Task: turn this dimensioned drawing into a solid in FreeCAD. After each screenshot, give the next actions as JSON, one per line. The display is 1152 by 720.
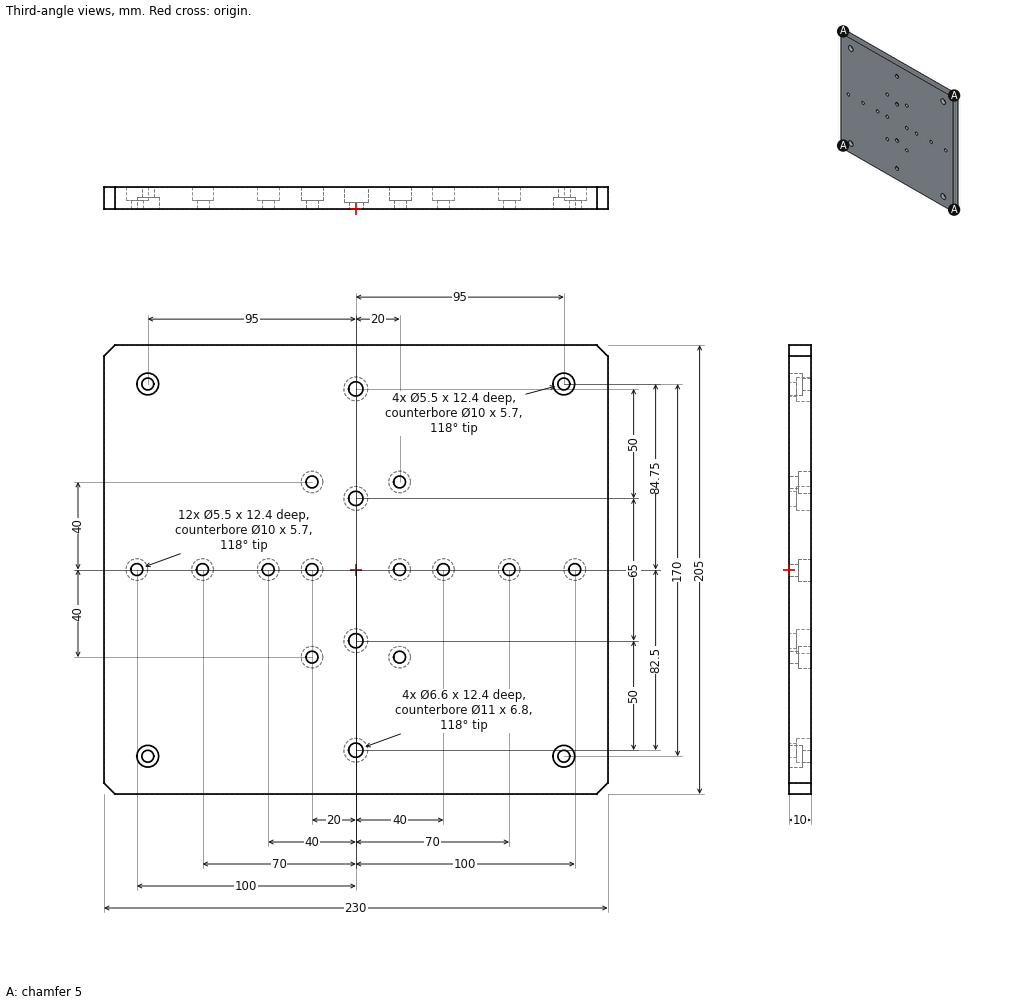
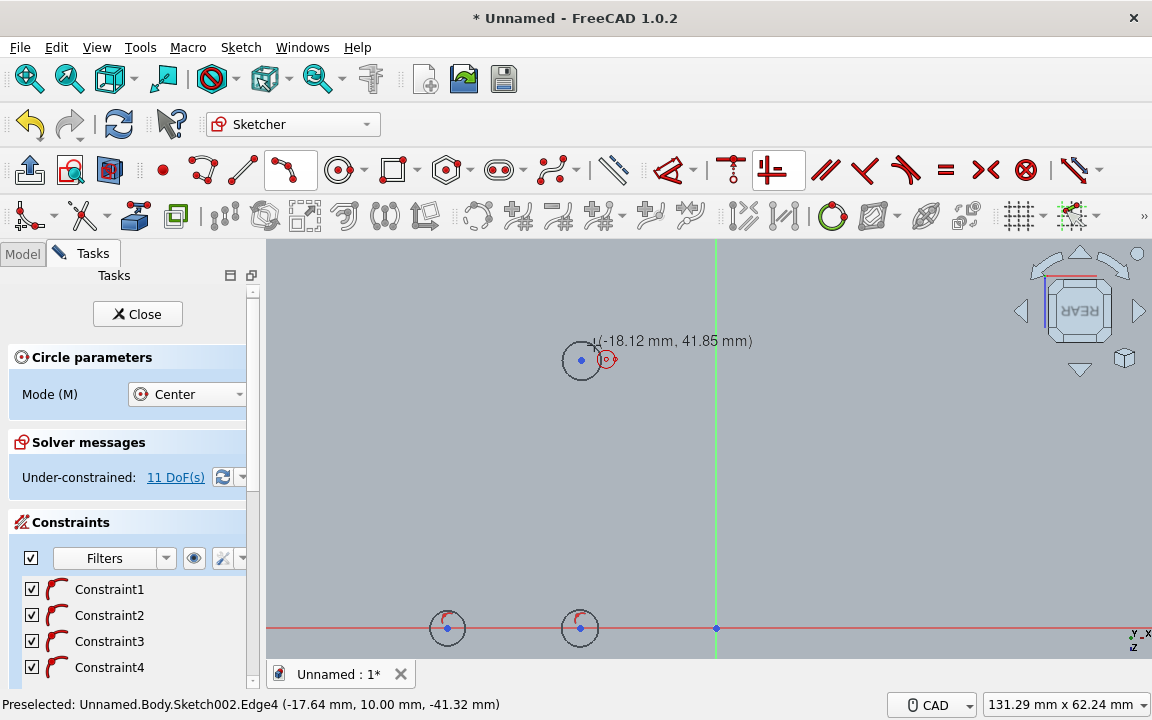
{"action": "scroll", "coordinate": [596, 345], "scroll_direction": "down", "scroll_amount": 5}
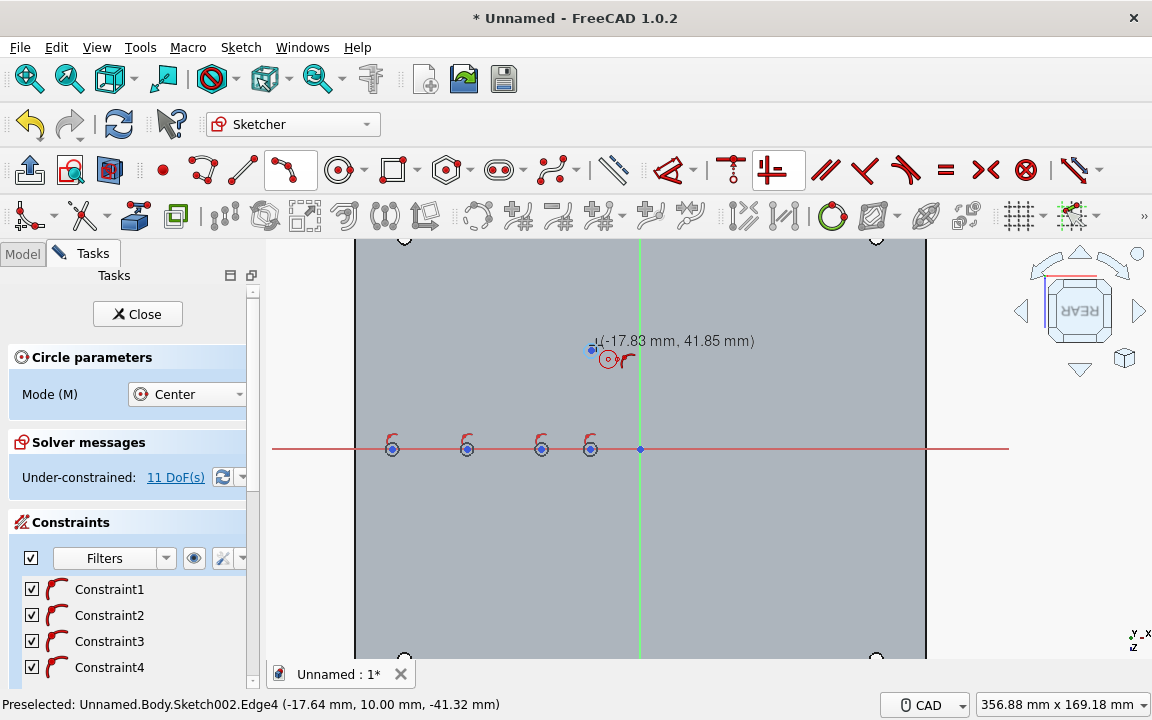
{"action": "scroll", "coordinate": [591, 549], "scroll_direction": "up", "scroll_amount": 7}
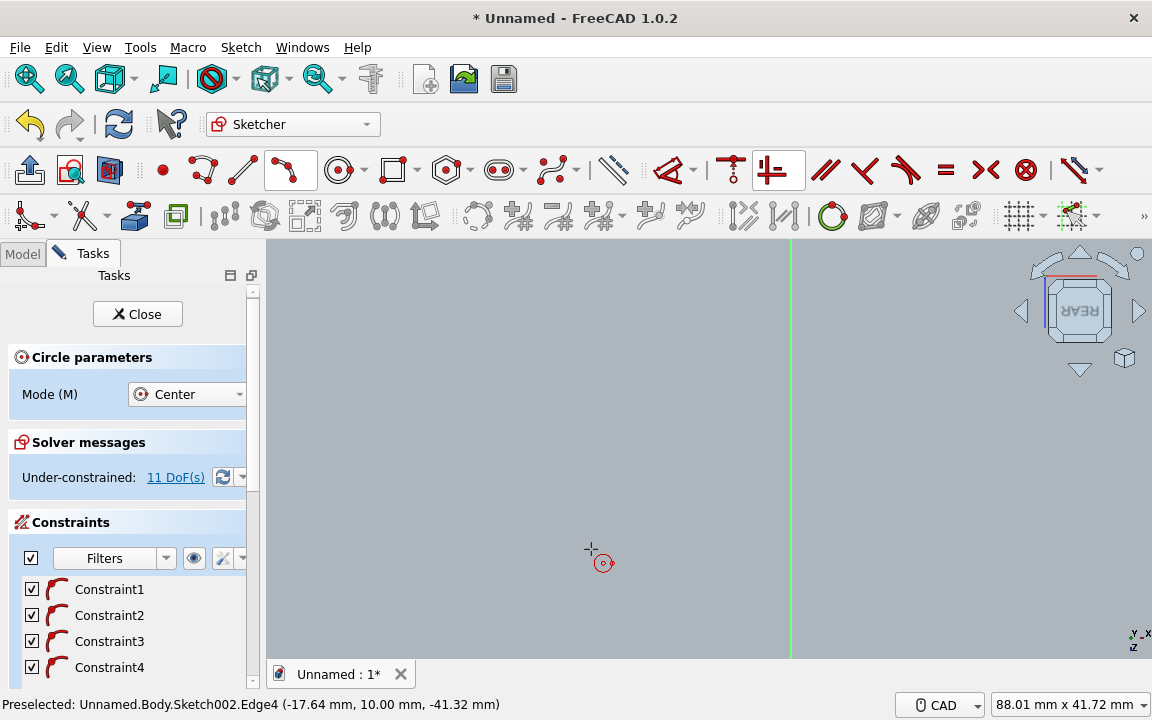
{"action": "scroll", "coordinate": [591, 549], "scroll_direction": "down", "scroll_amount": 7}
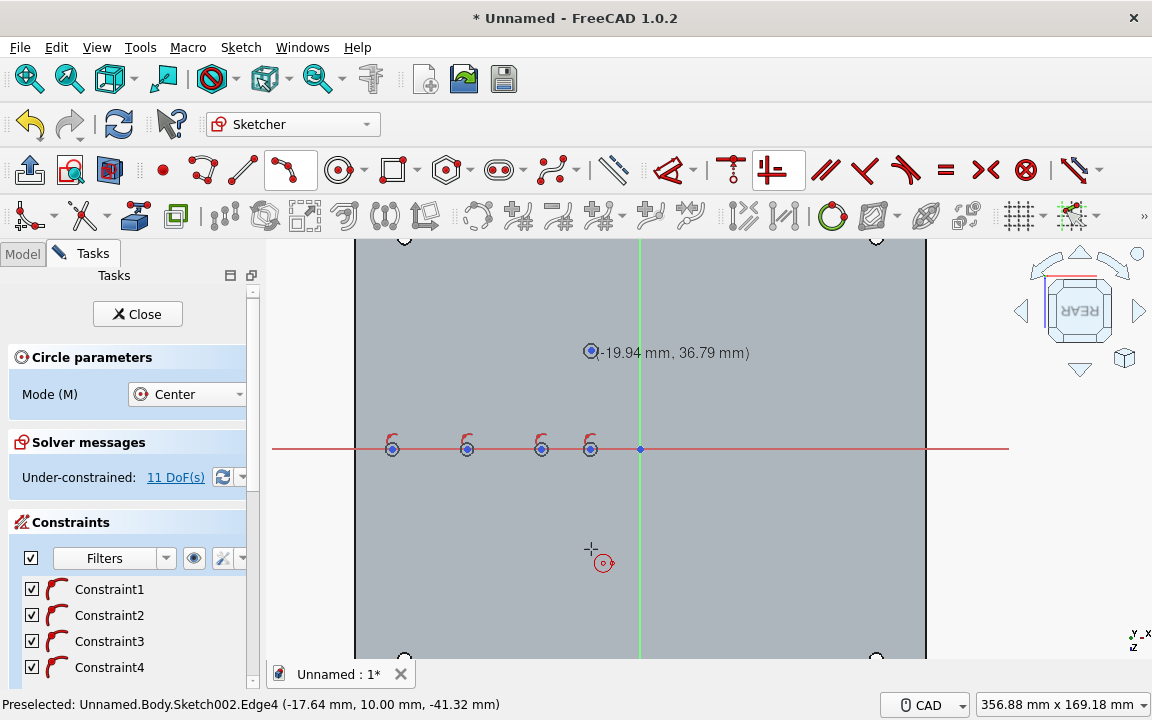
{"action": "left_click", "coordinate": [591, 549]}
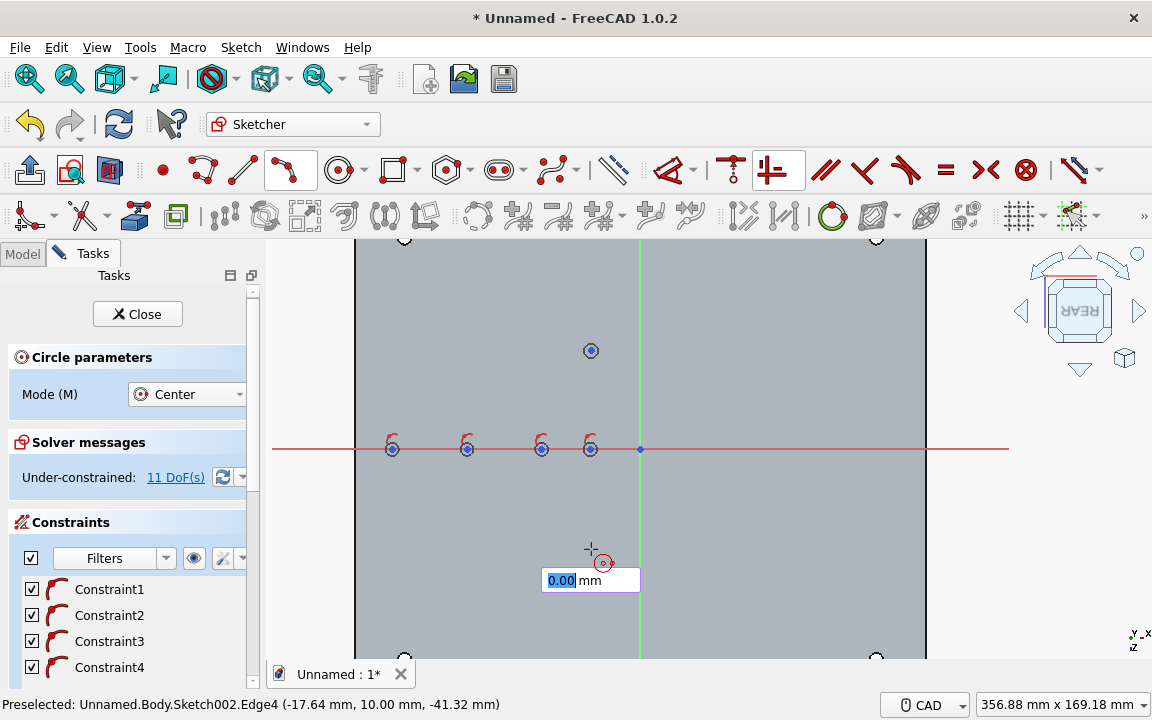
{"action": "scroll", "coordinate": [596, 544], "scroll_direction": "up", "scroll_amount": 5}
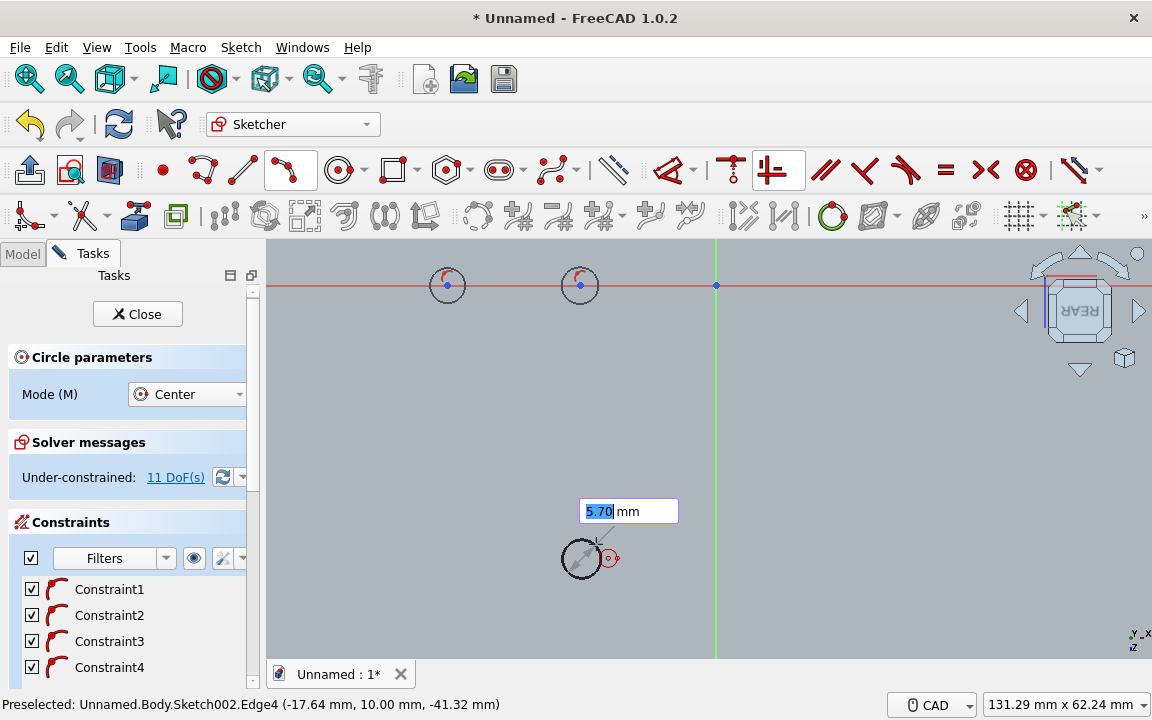
{"action": "left_click", "coordinate": [594, 542]}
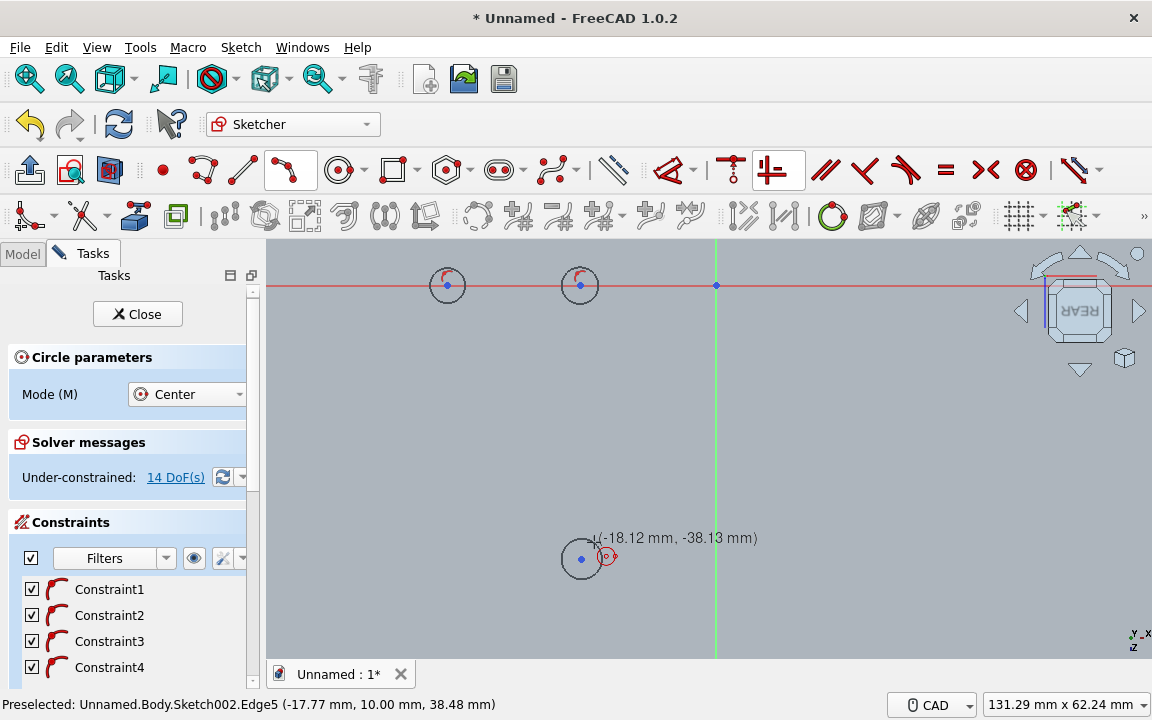
{"action": "scroll", "coordinate": [851, 556], "scroll_direction": "up", "scroll_amount": 2}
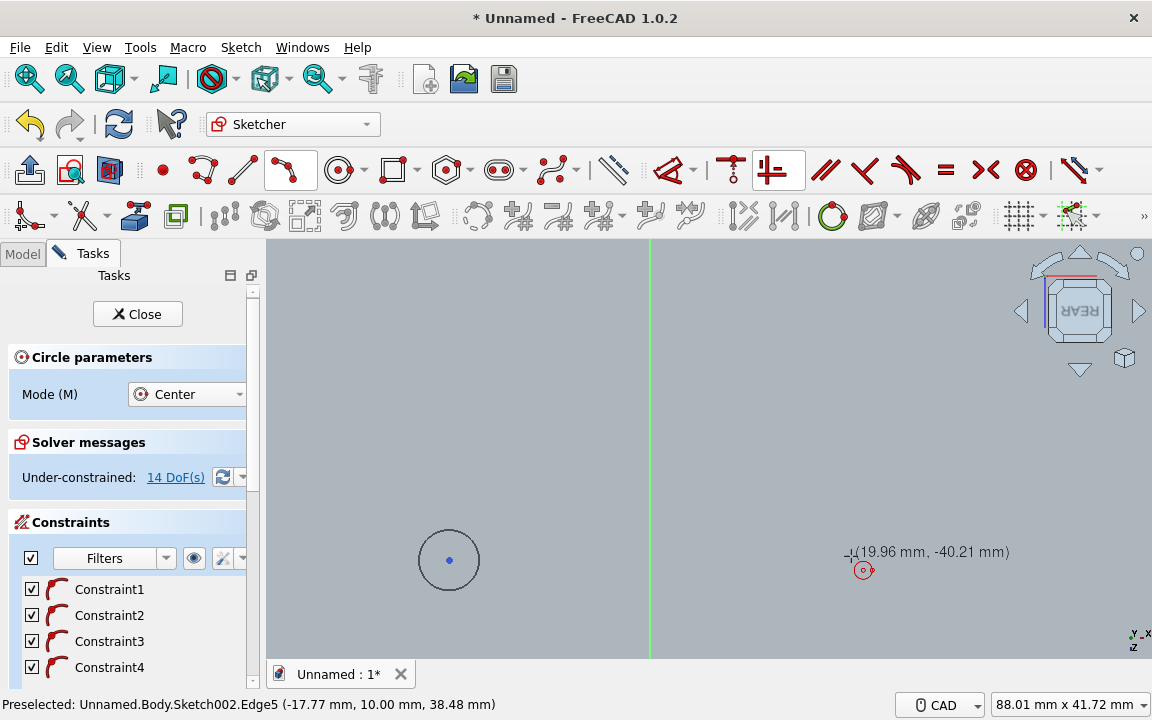
{"action": "scroll", "coordinate": [637, 546], "scroll_direction": "down", "scroll_amount": 7}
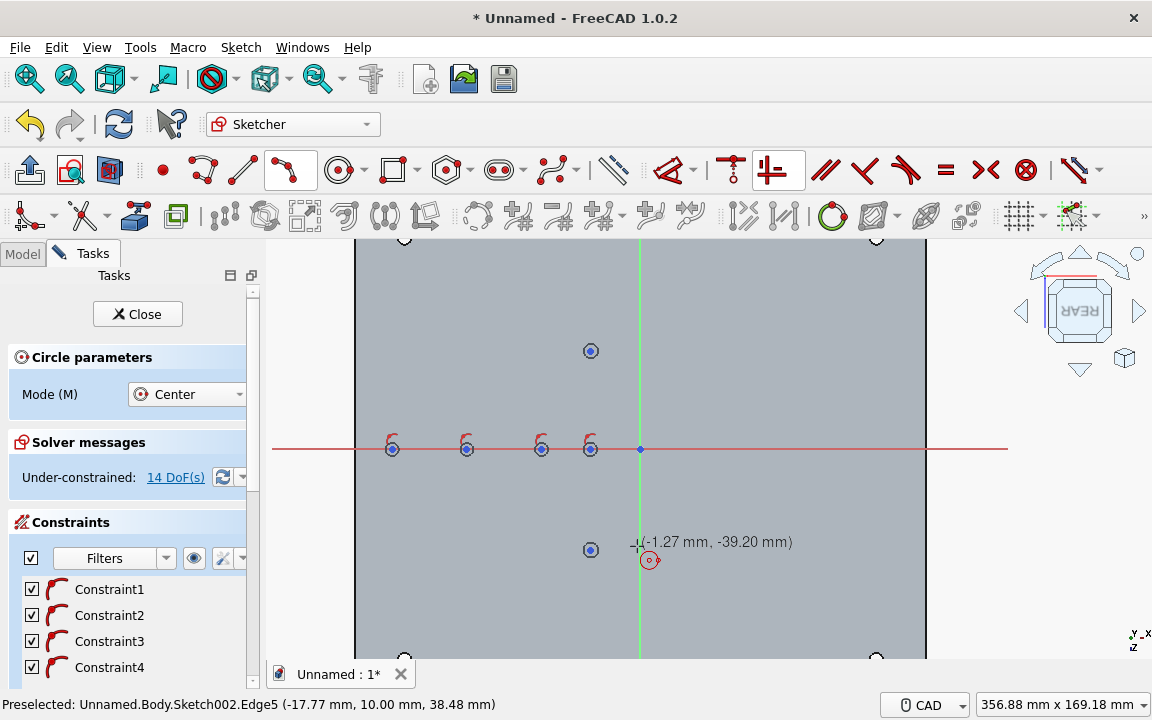
{"action": "left_click", "coordinate": [690, 549]}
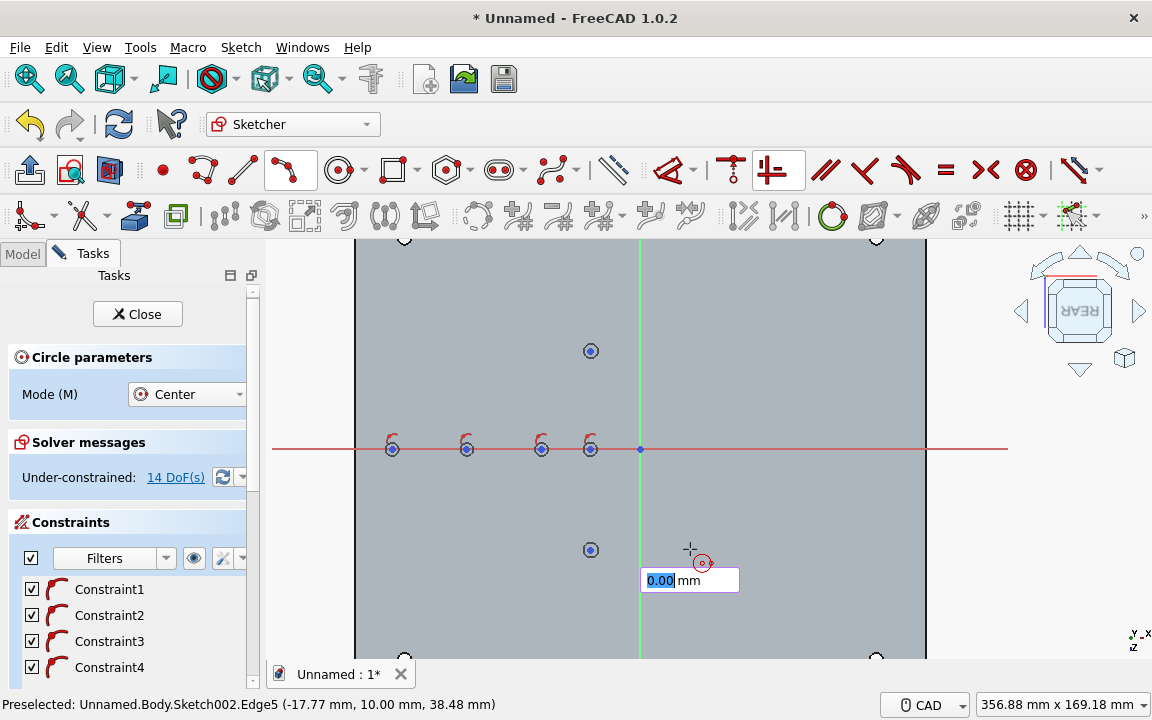
{"action": "scroll", "coordinate": [695, 544], "scroll_direction": "up", "scroll_amount": 5}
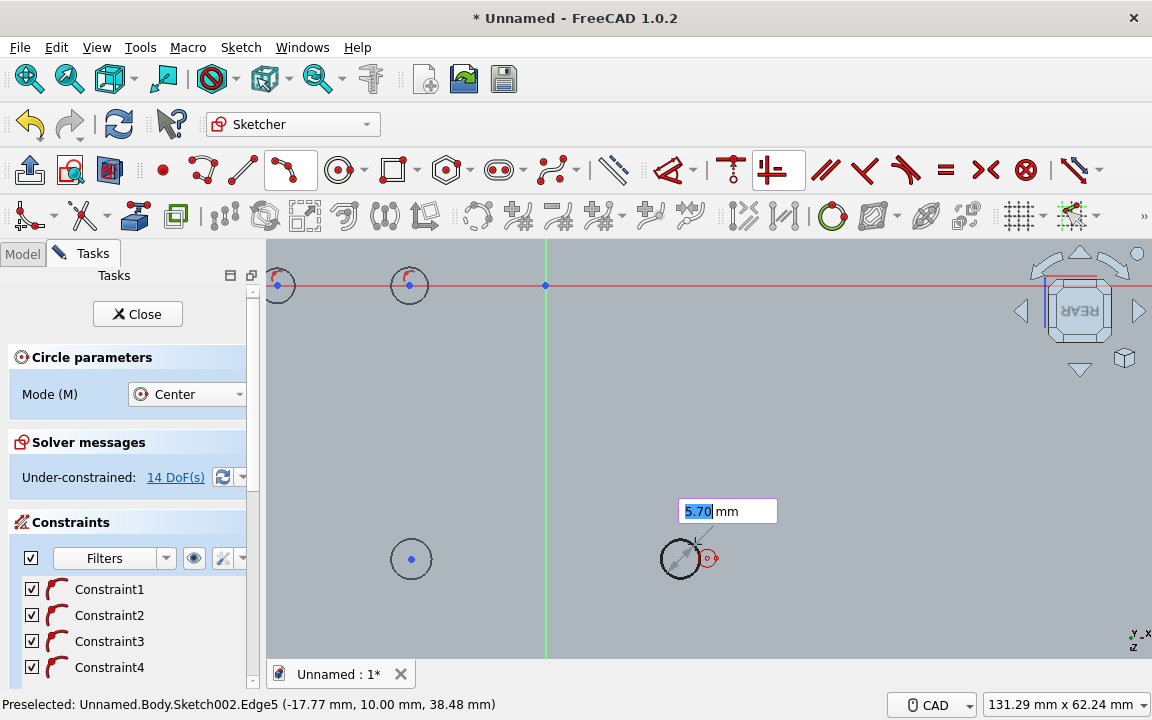
{"action": "left_click", "coordinate": [694, 543]}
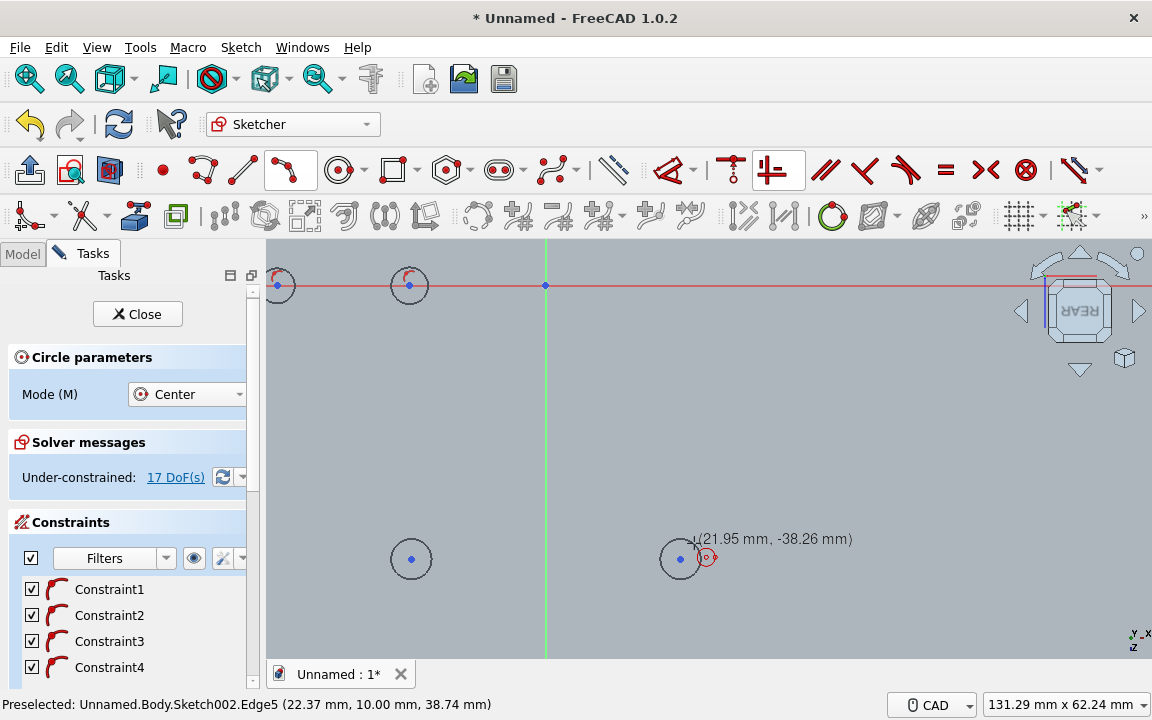
{"action": "scroll", "coordinate": [816, 286], "scroll_direction": "up", "scroll_amount": 2}